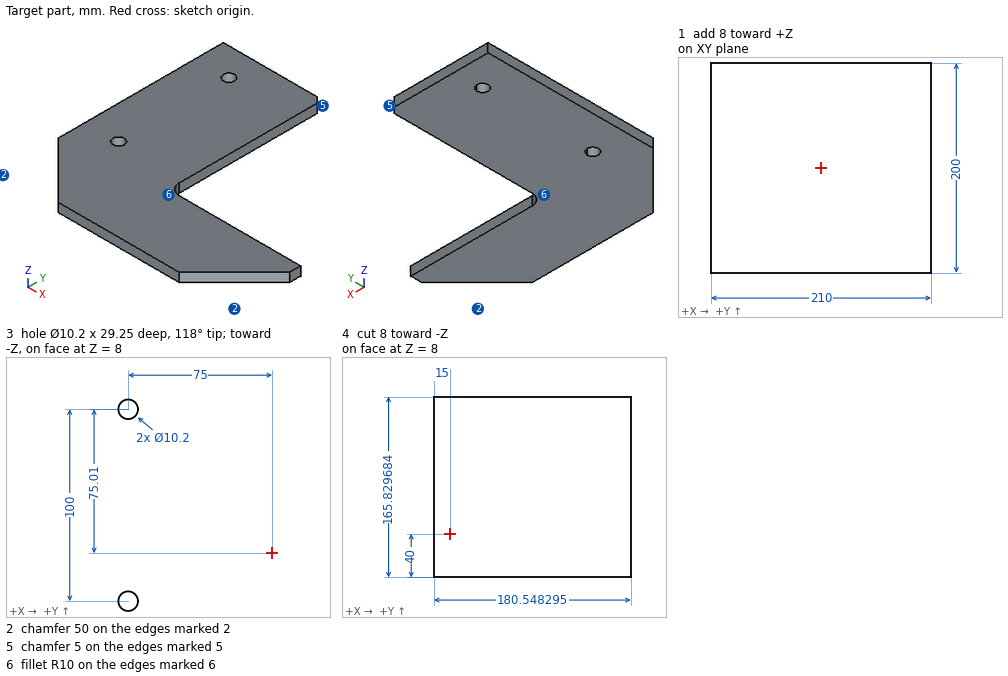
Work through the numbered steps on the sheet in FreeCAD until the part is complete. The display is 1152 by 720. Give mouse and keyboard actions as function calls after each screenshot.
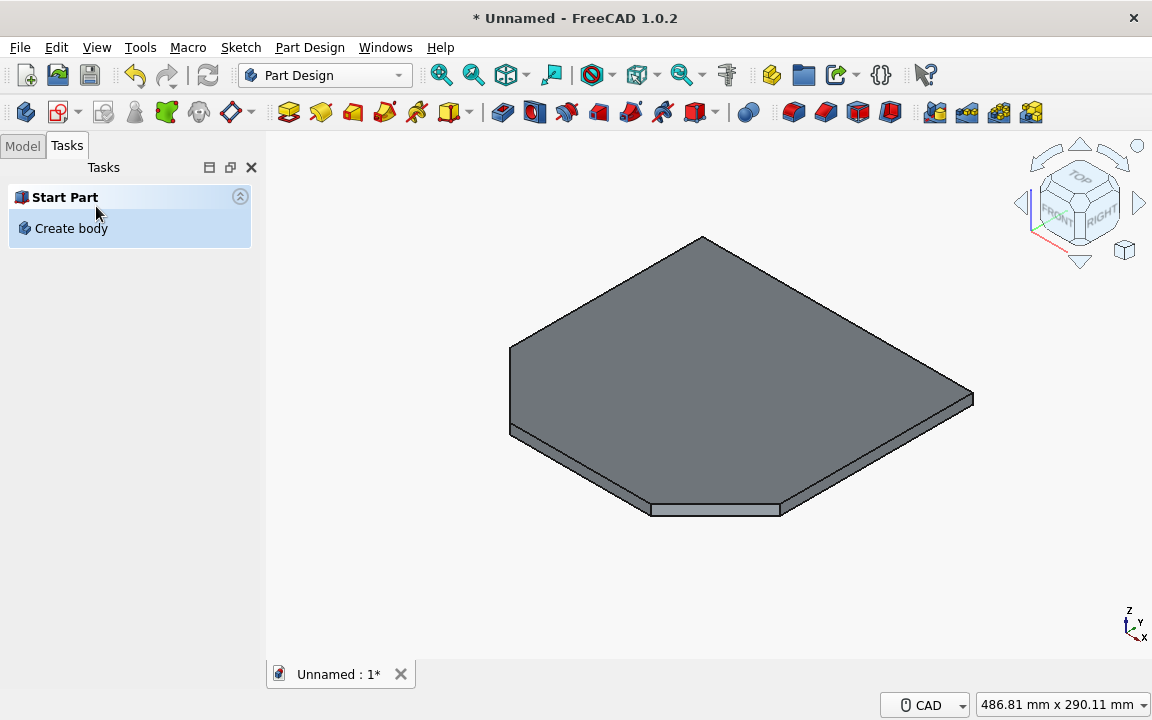
click(709, 388)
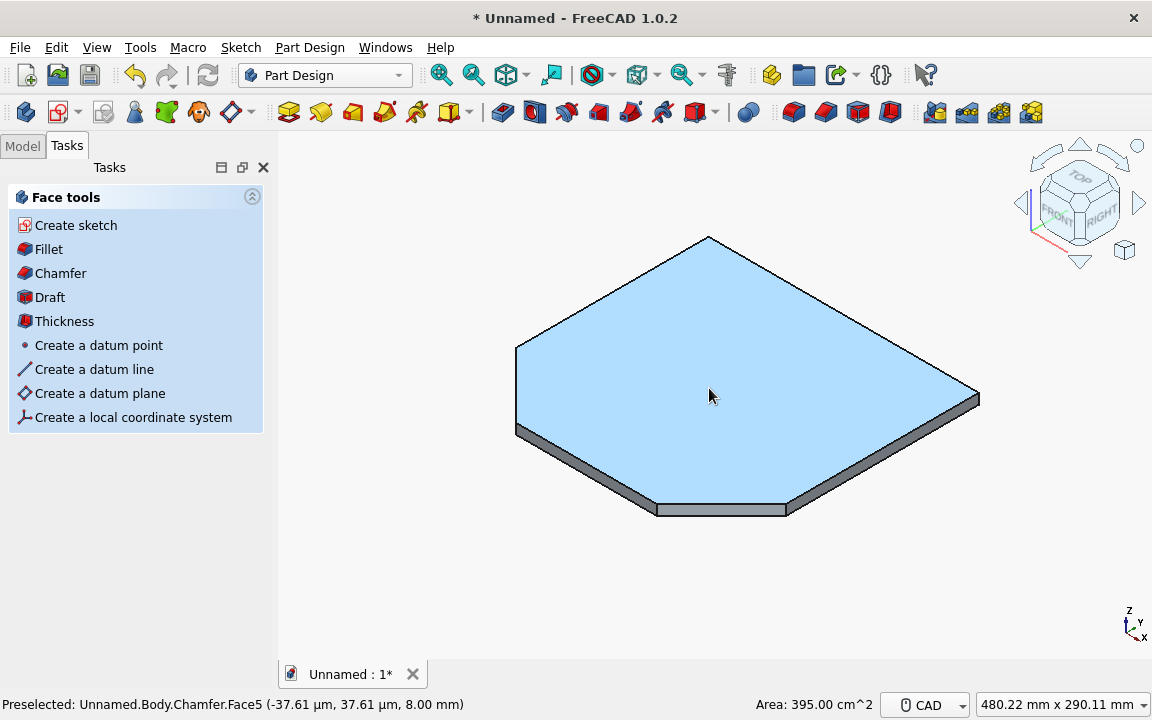
click(58, 112)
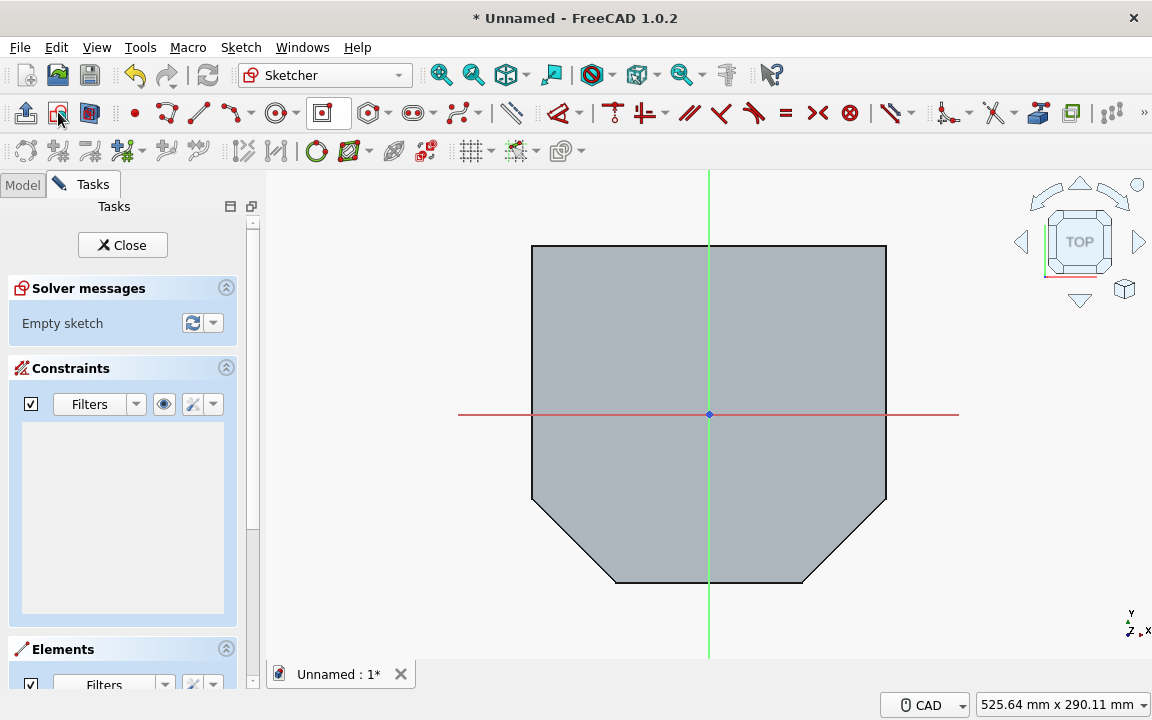
scroll(644, 287, up, 2)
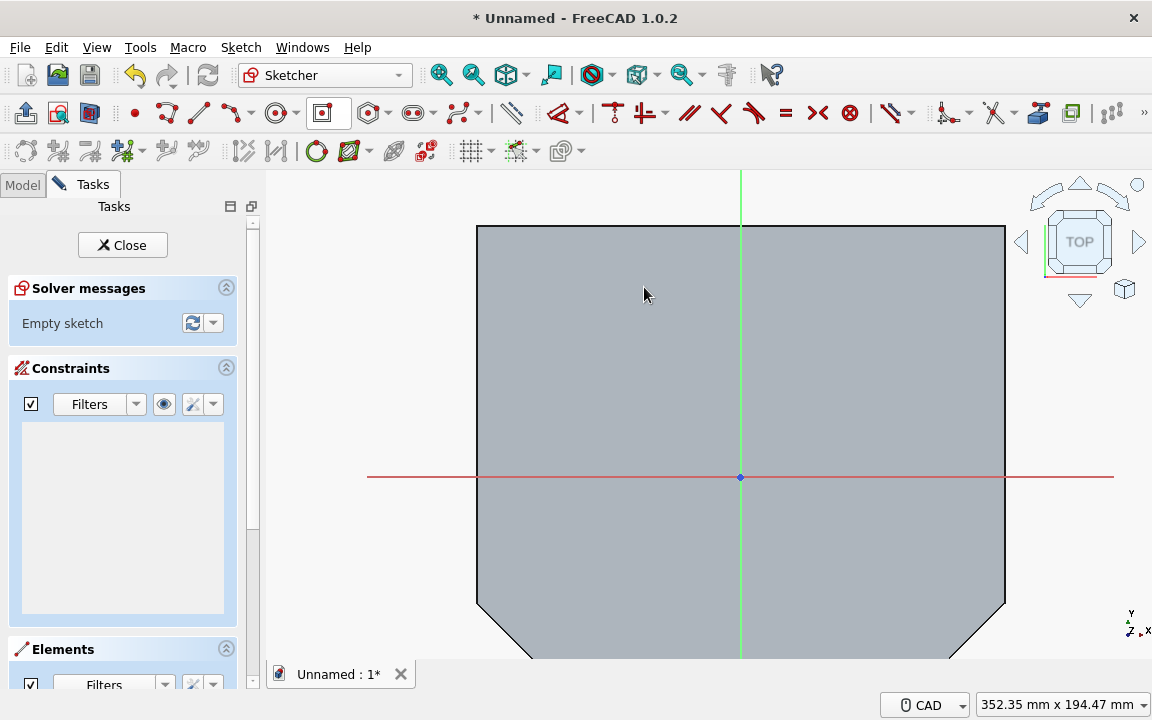
key(g)
key(c)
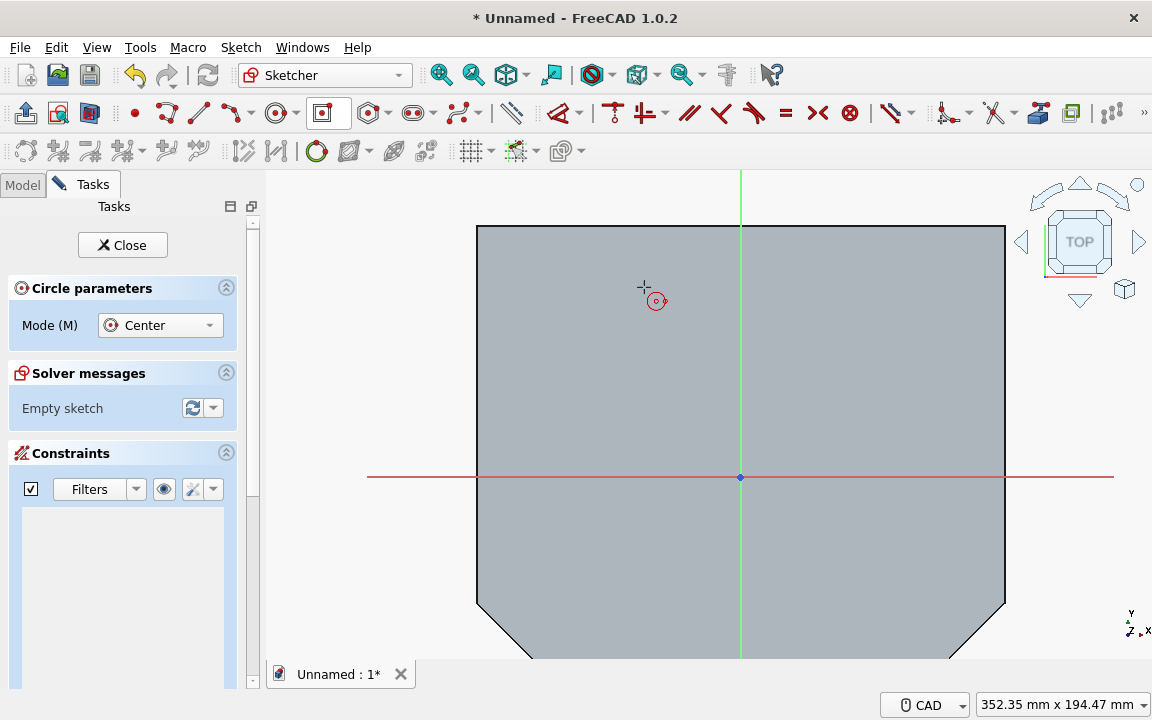
scroll(552, 288, up, 3)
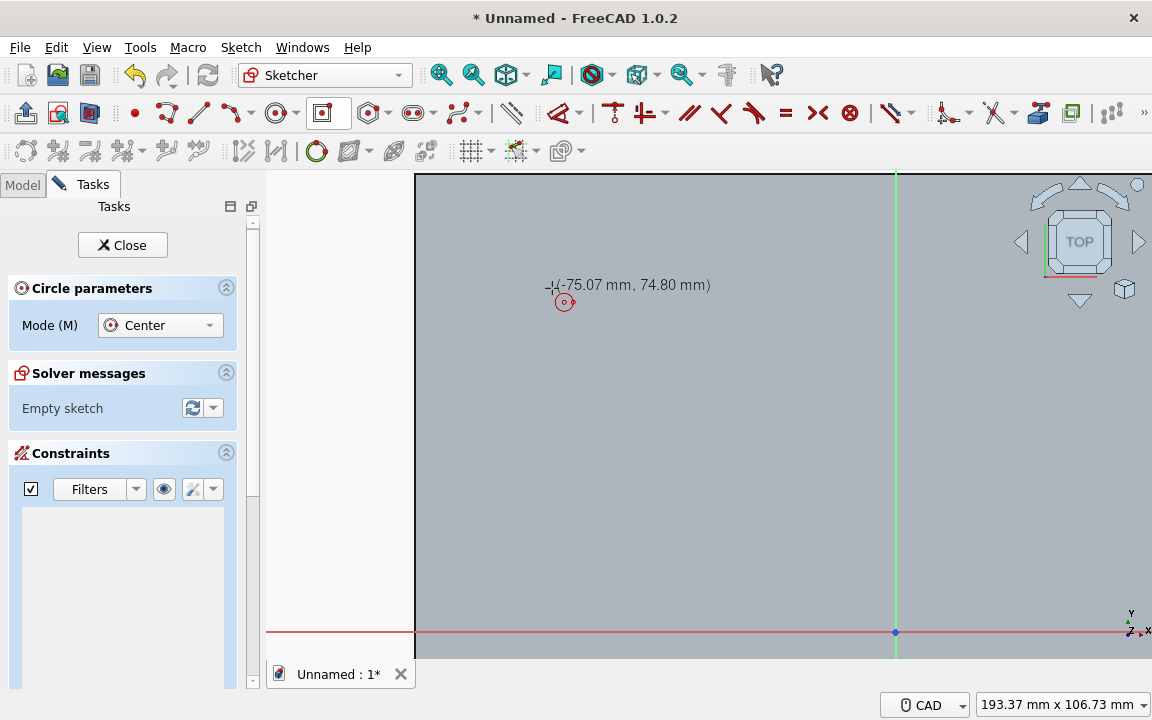
click(552, 289)
click(569, 272)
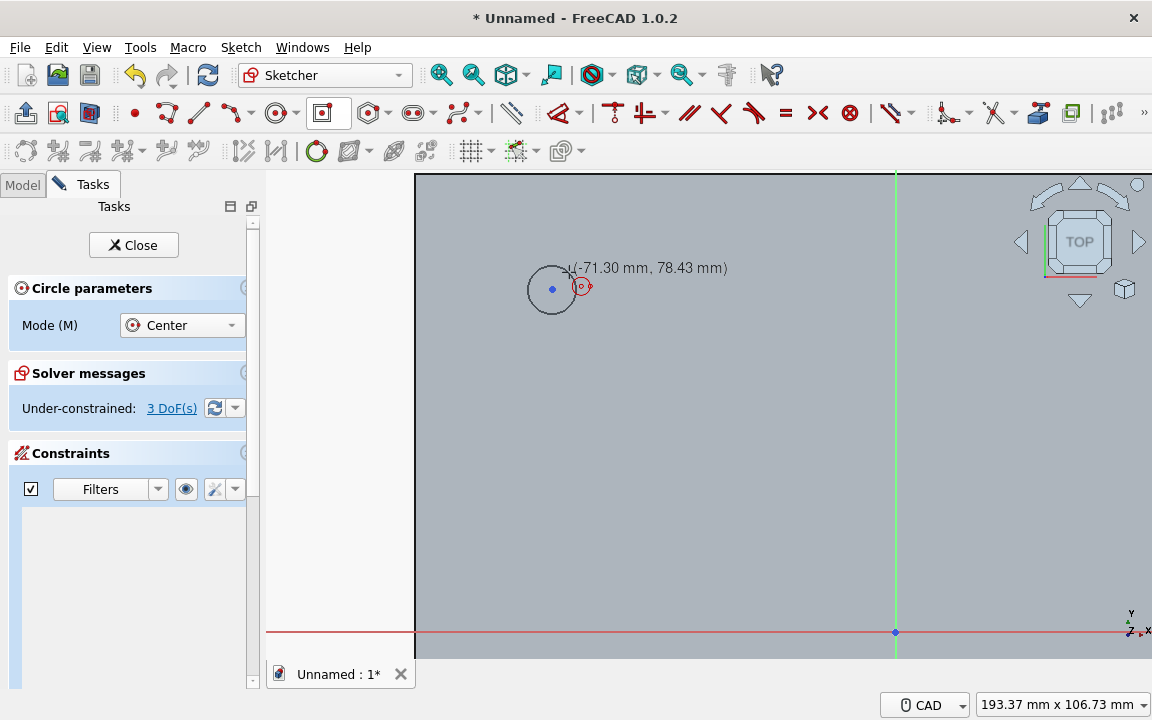
scroll(553, 289, down, 3)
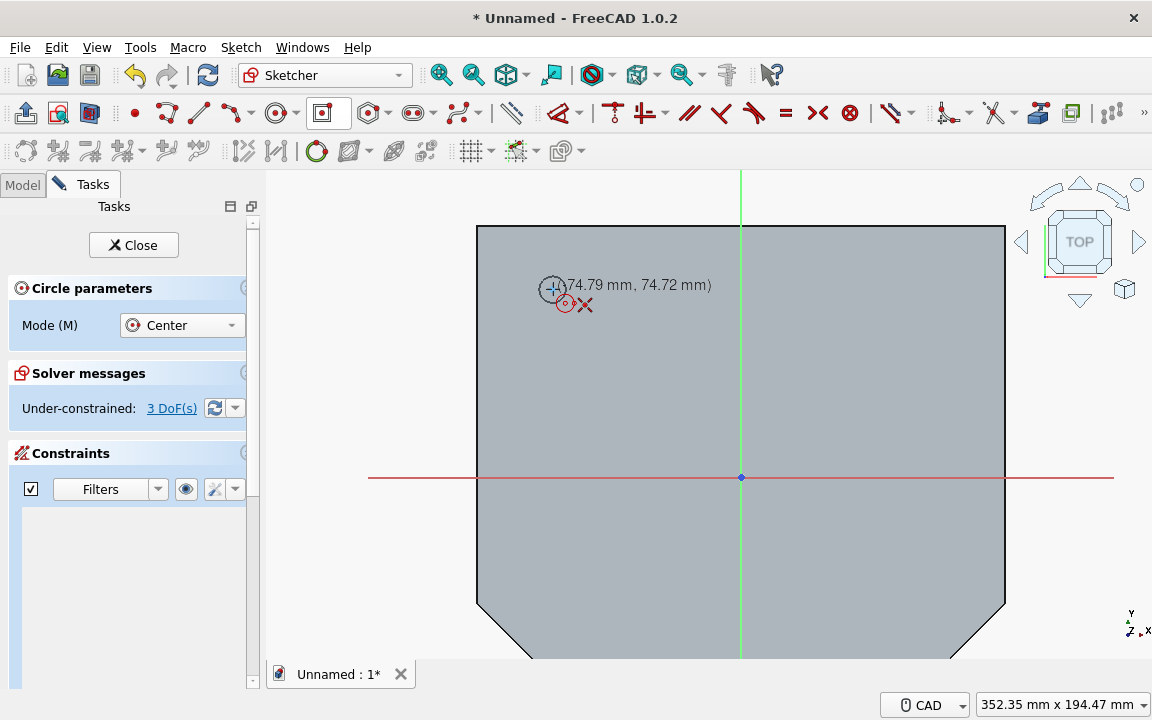
scroll(553, 540, up, 3)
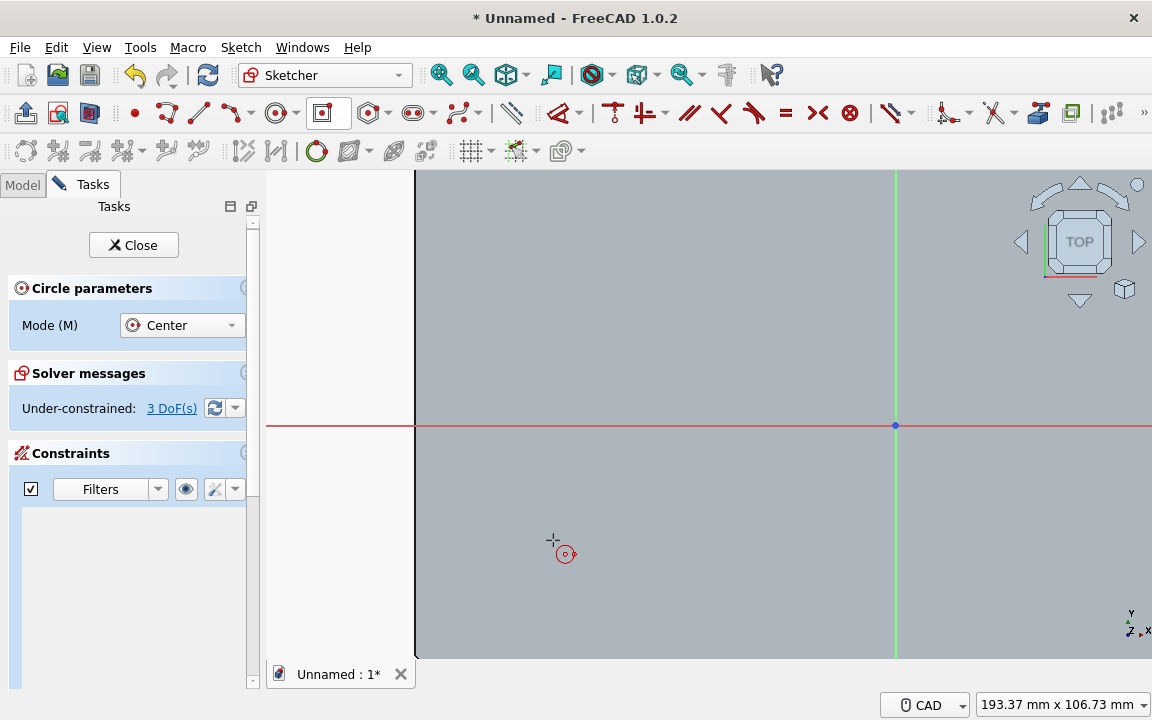
click(552, 540)
click(569, 524)
key(Escape)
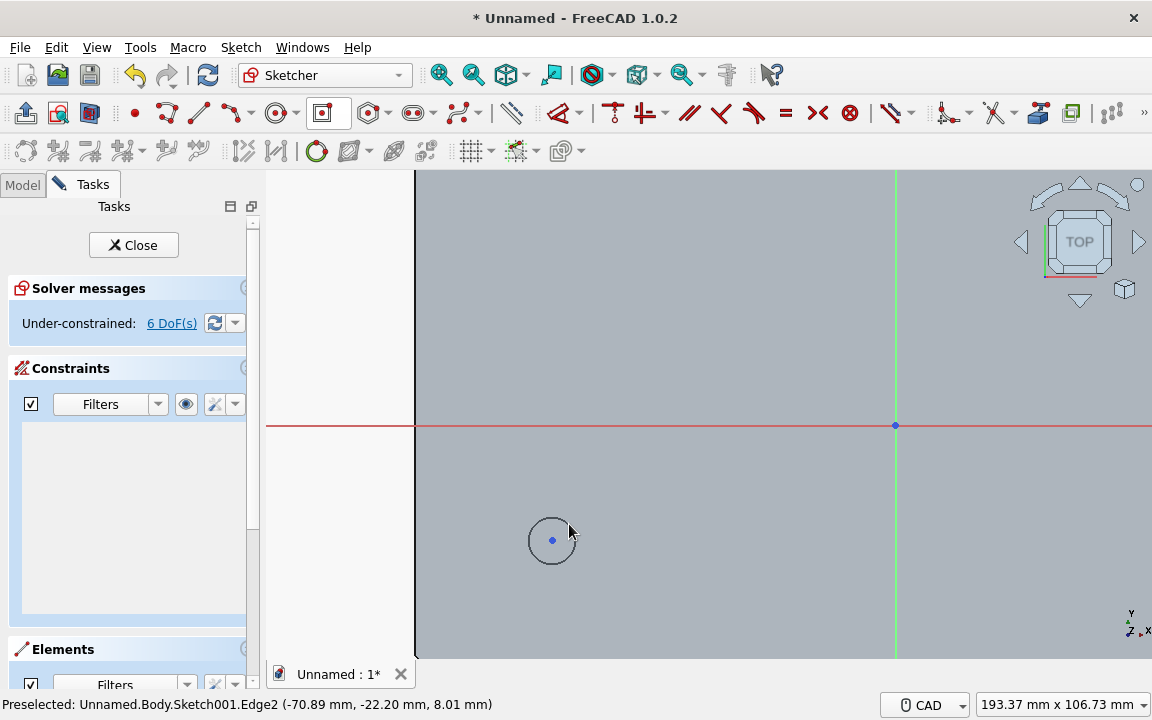
scroll(553, 540, down, 3)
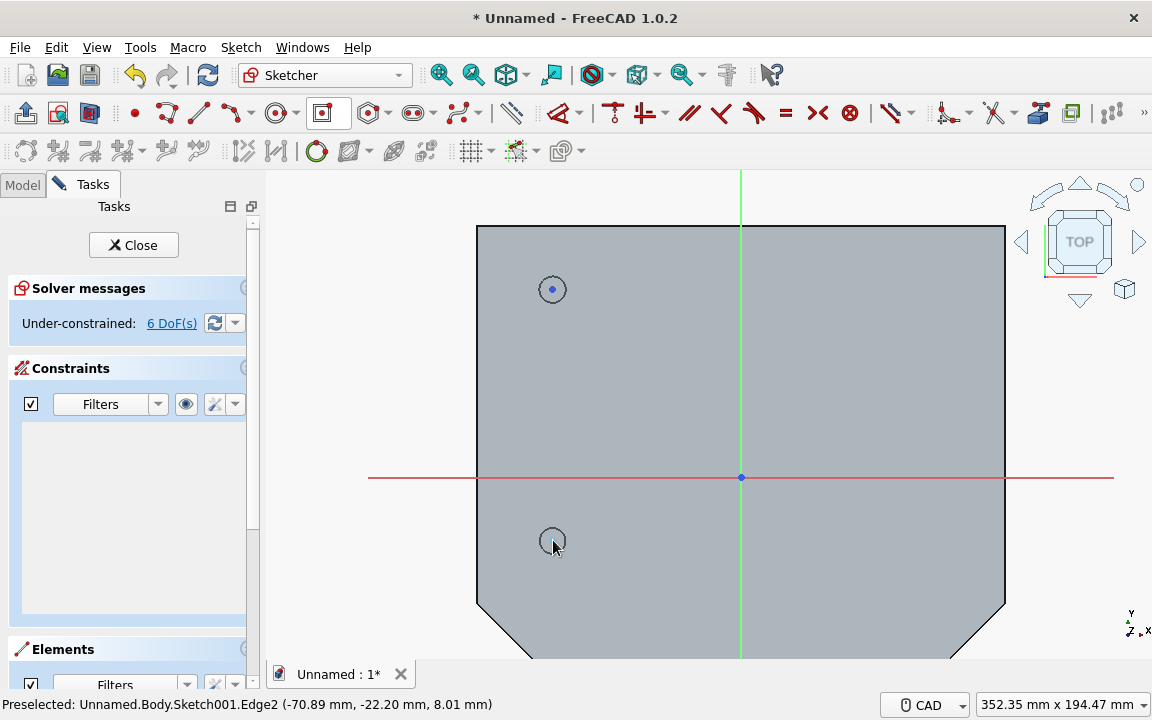
click(562, 280)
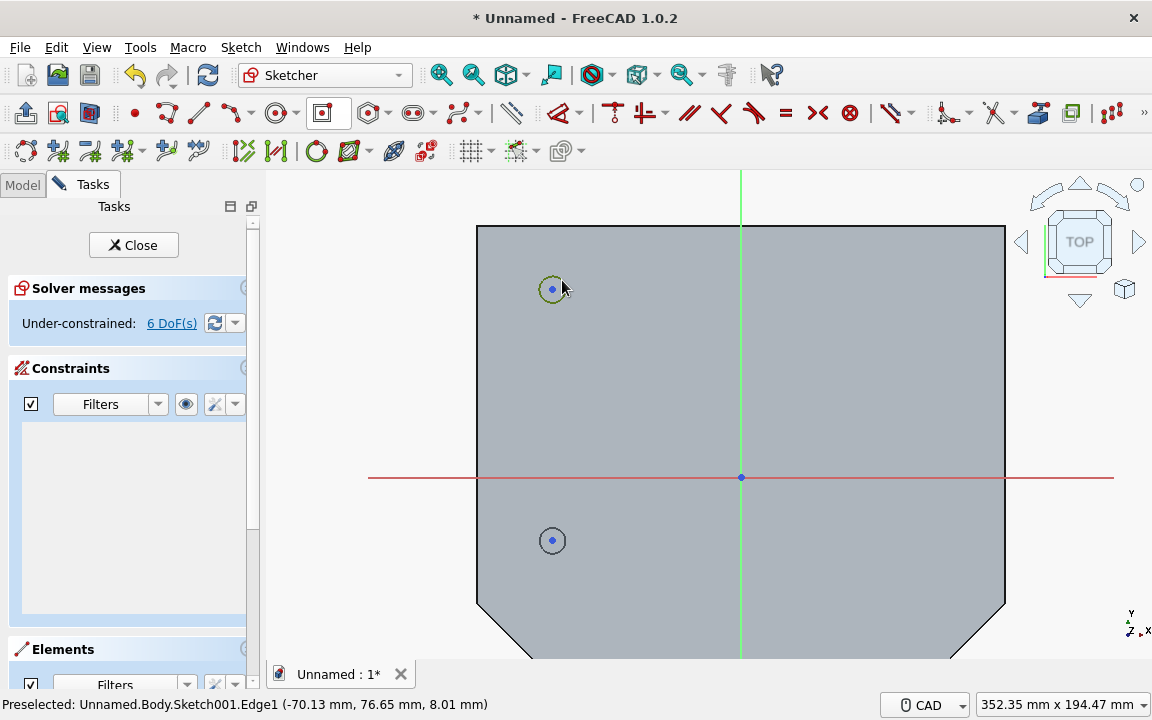
click(562, 532)